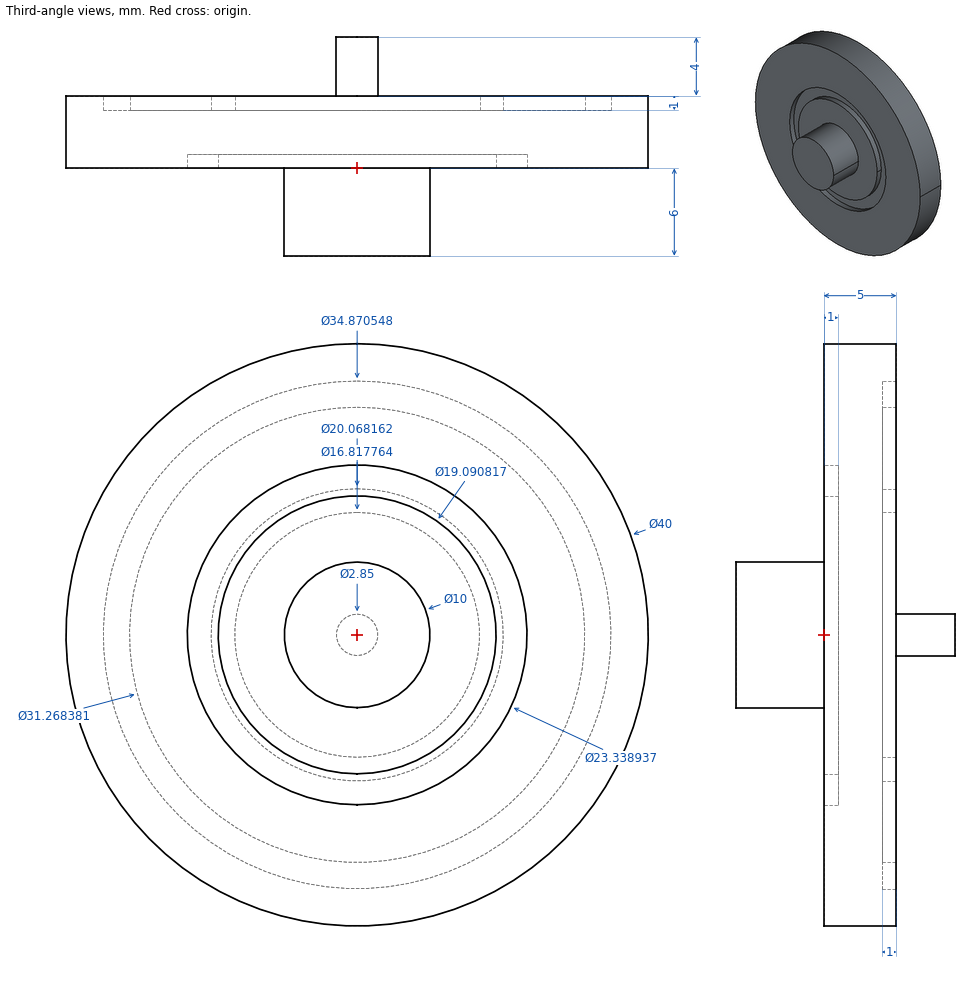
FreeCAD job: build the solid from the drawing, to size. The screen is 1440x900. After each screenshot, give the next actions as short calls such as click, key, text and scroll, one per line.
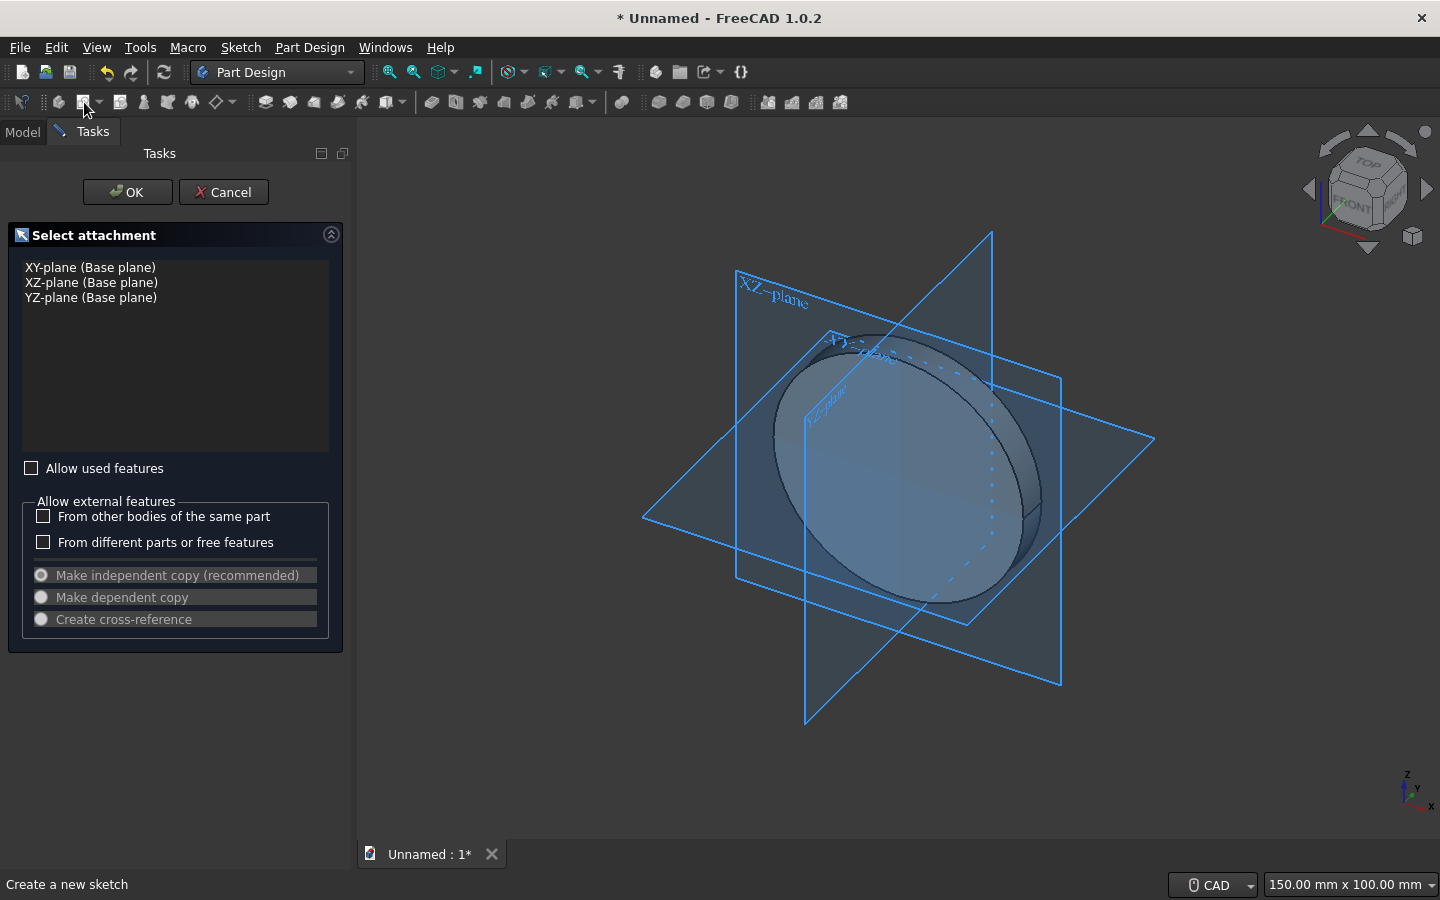
click(82, 282)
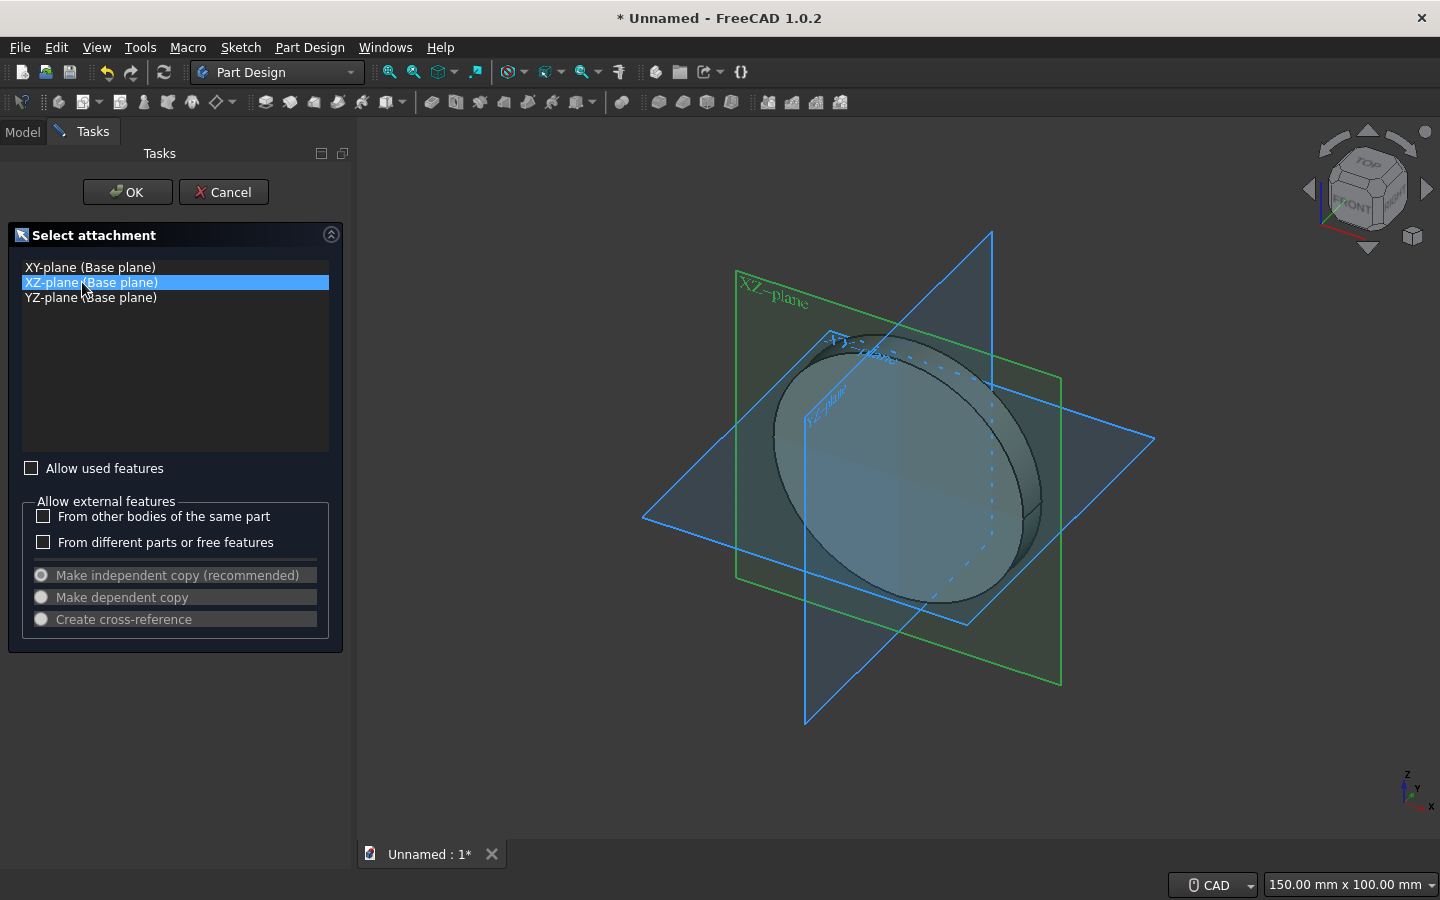
click(128, 192)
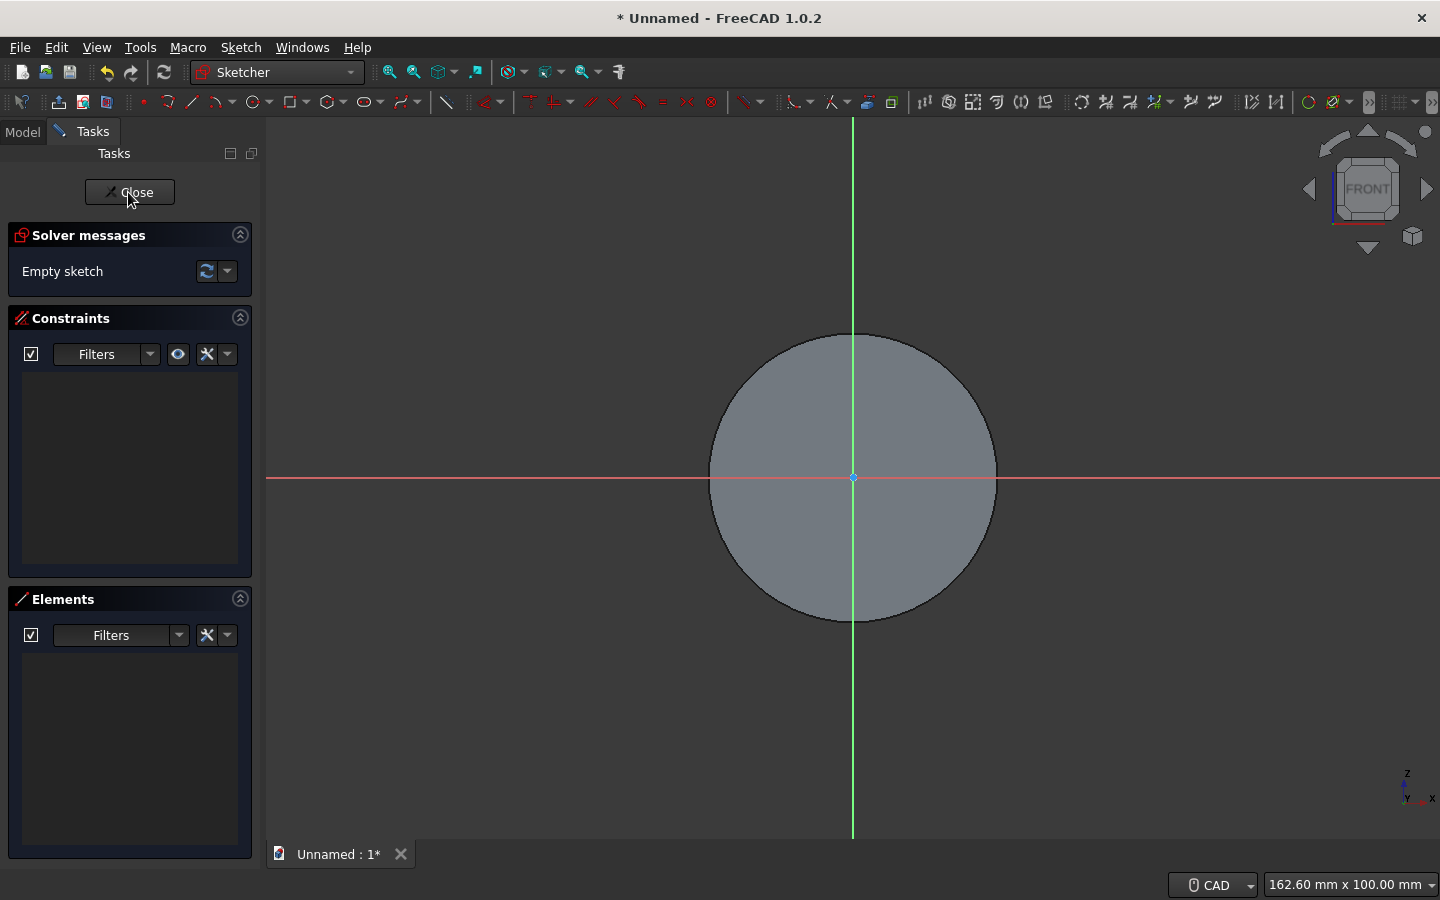
scroll(867, 478, up, 9)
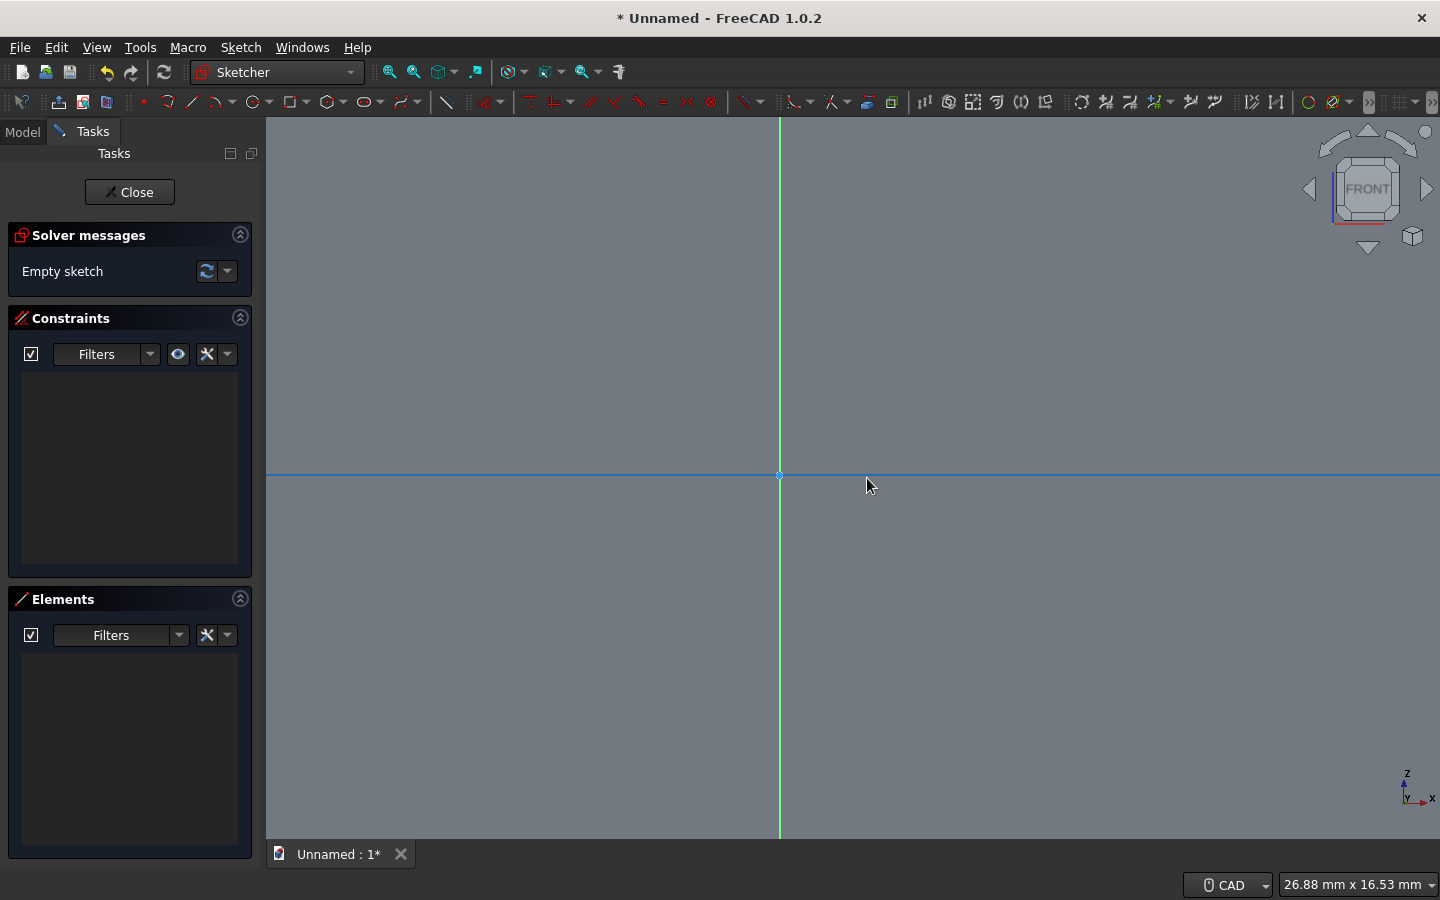
key(g)
key(c)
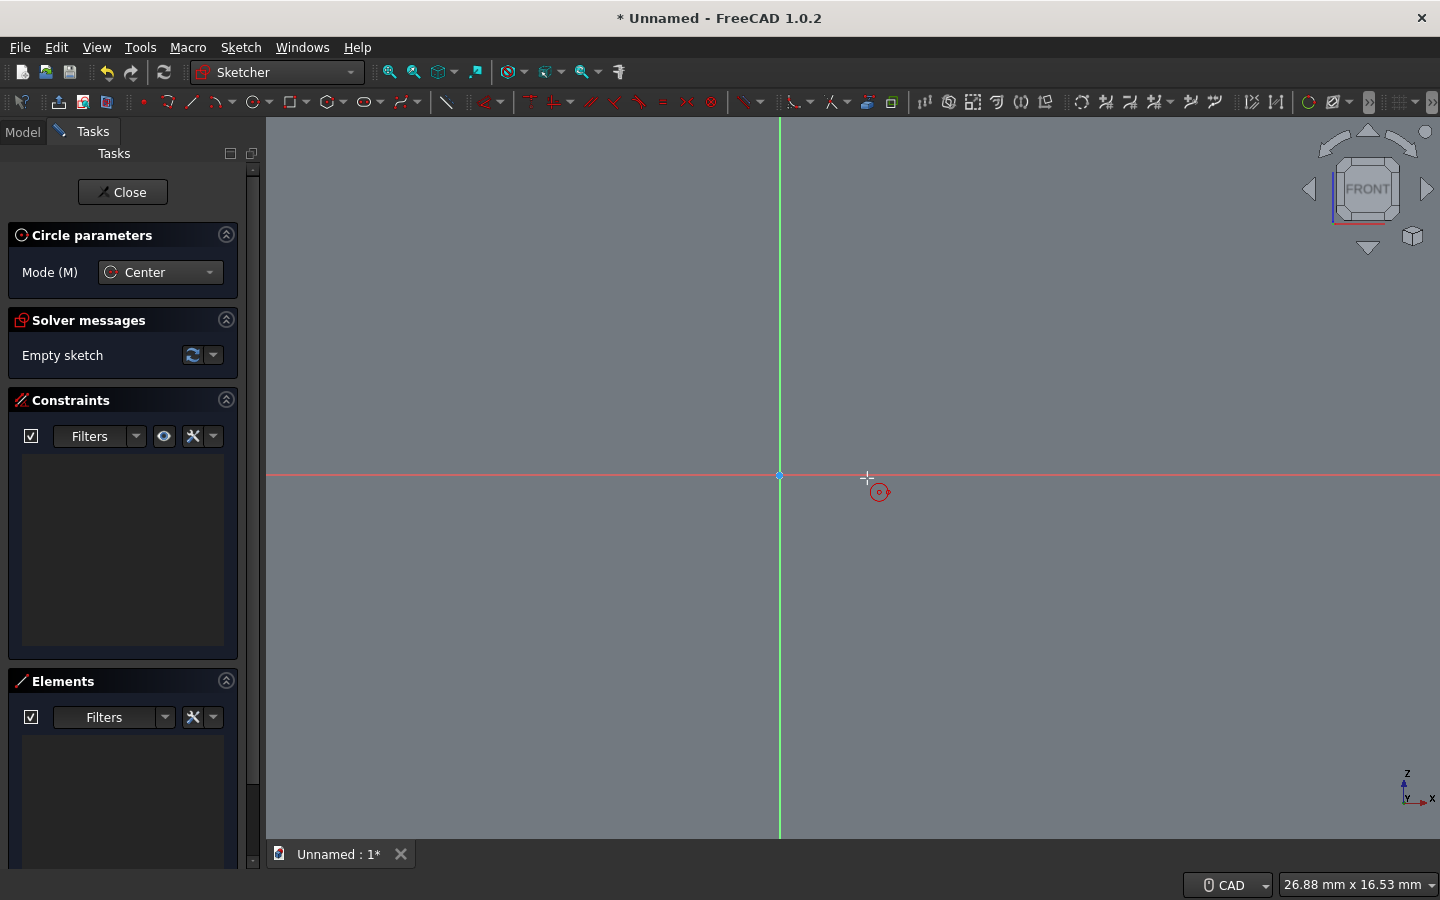
click(780, 475)
click(934, 321)
key(Escape)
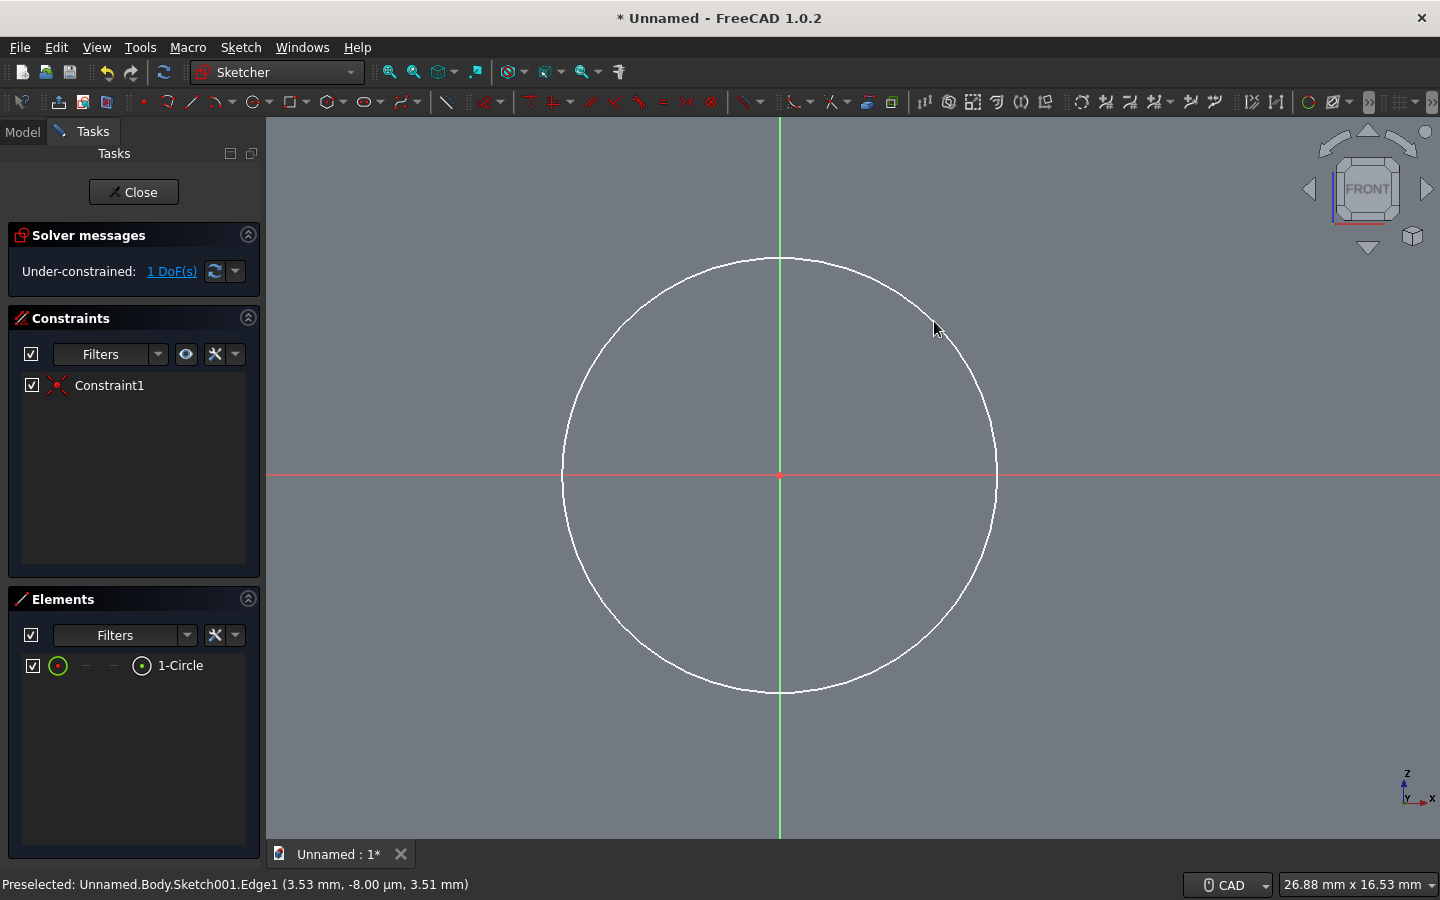
key(d)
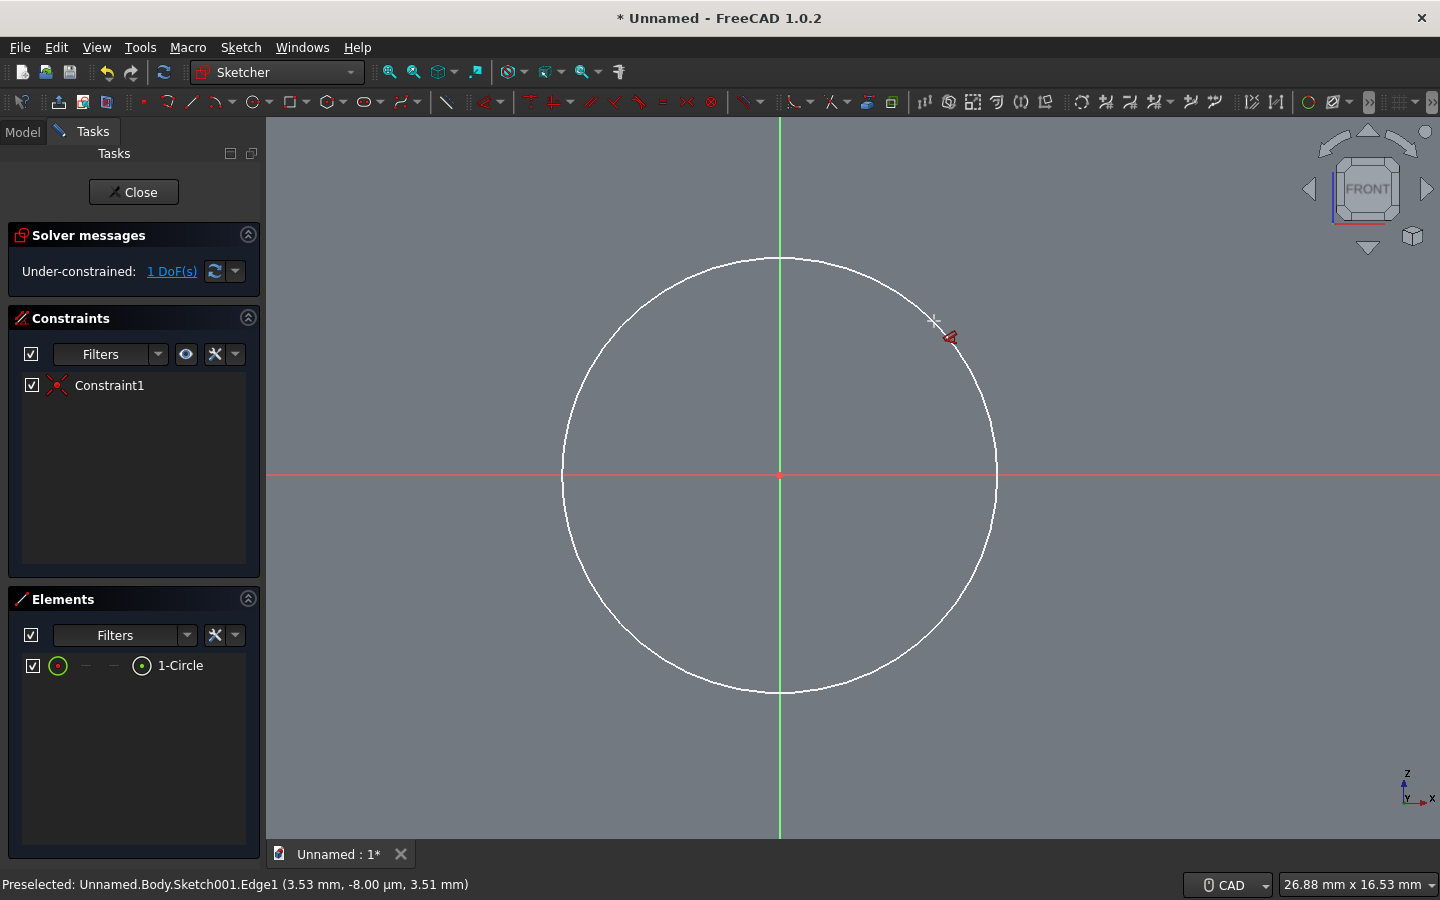
click(933, 321)
click(956, 298)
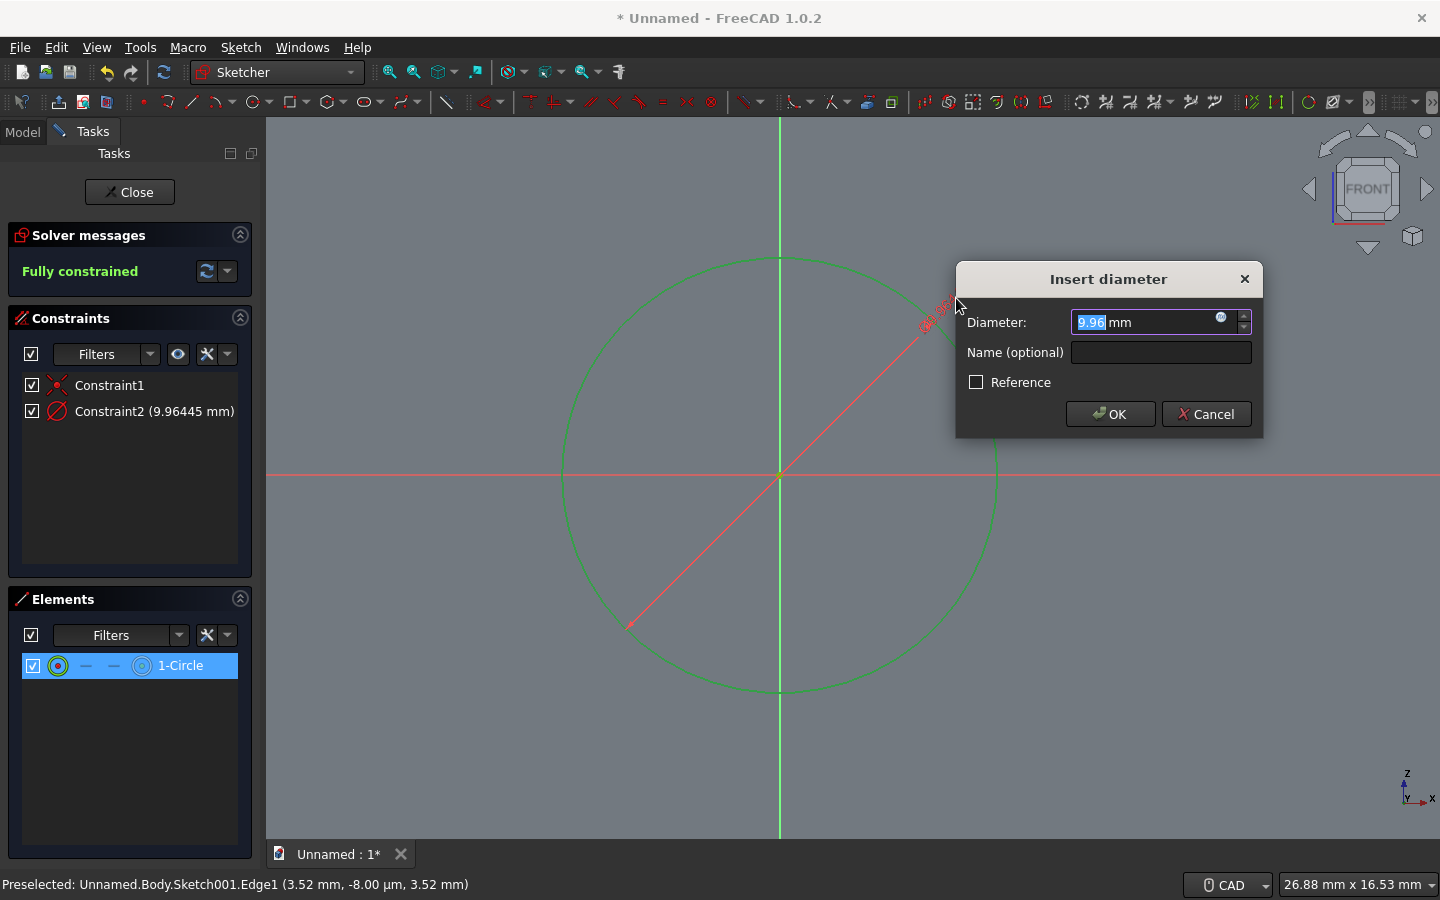
text(10)
key(Return)
key(Escape)